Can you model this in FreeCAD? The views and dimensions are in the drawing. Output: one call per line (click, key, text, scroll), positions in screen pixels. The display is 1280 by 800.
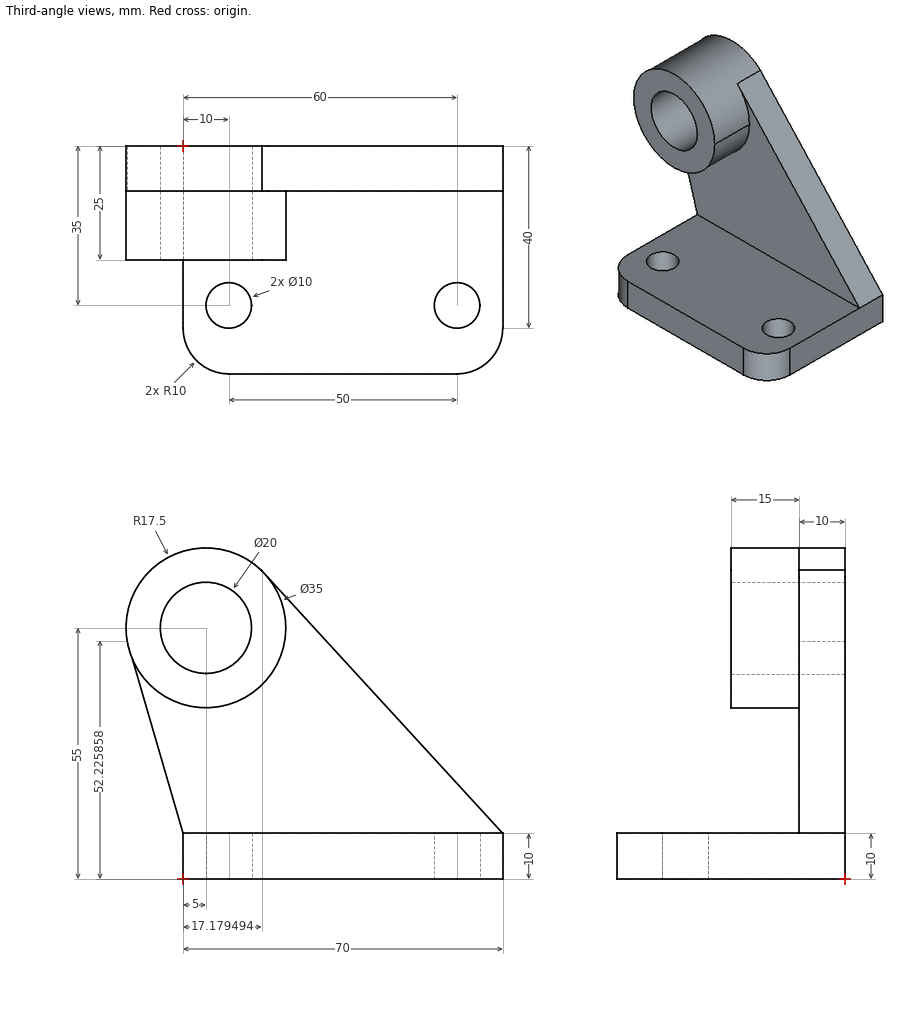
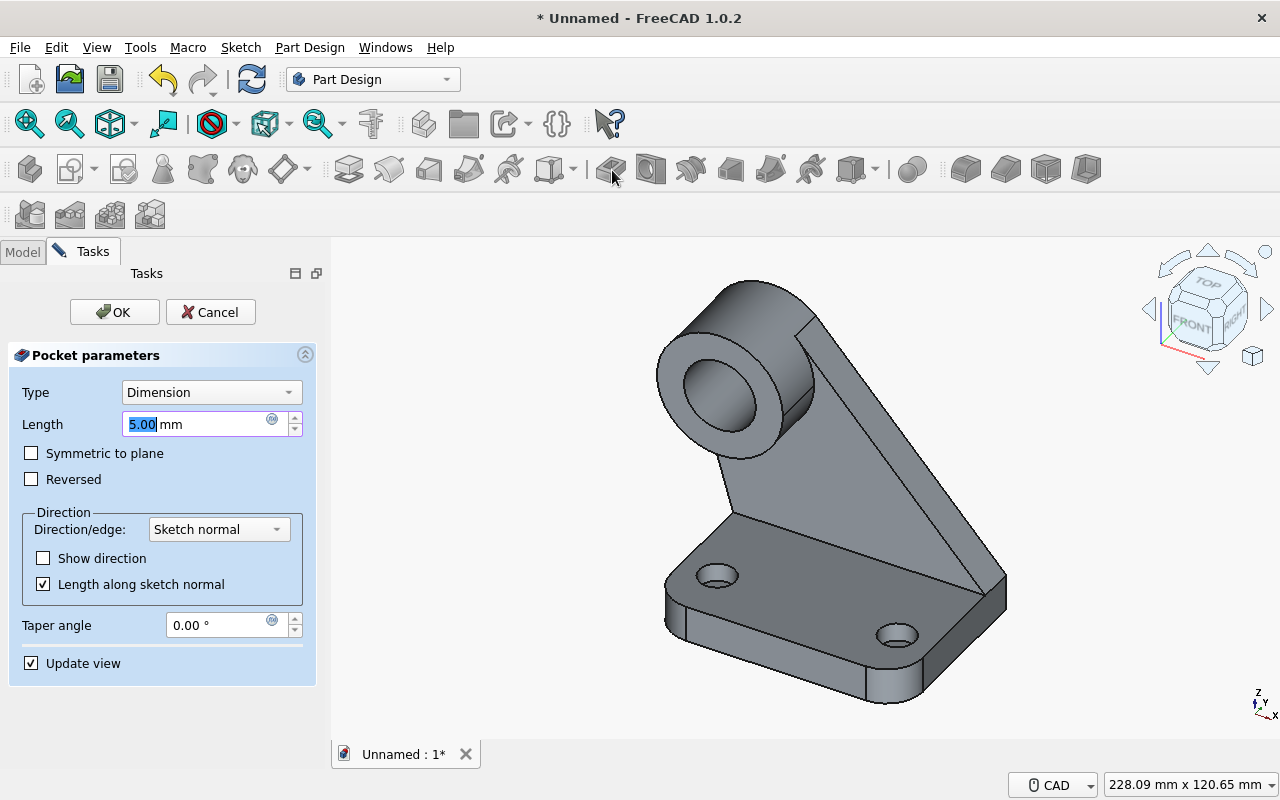
text(10)
key(Tab)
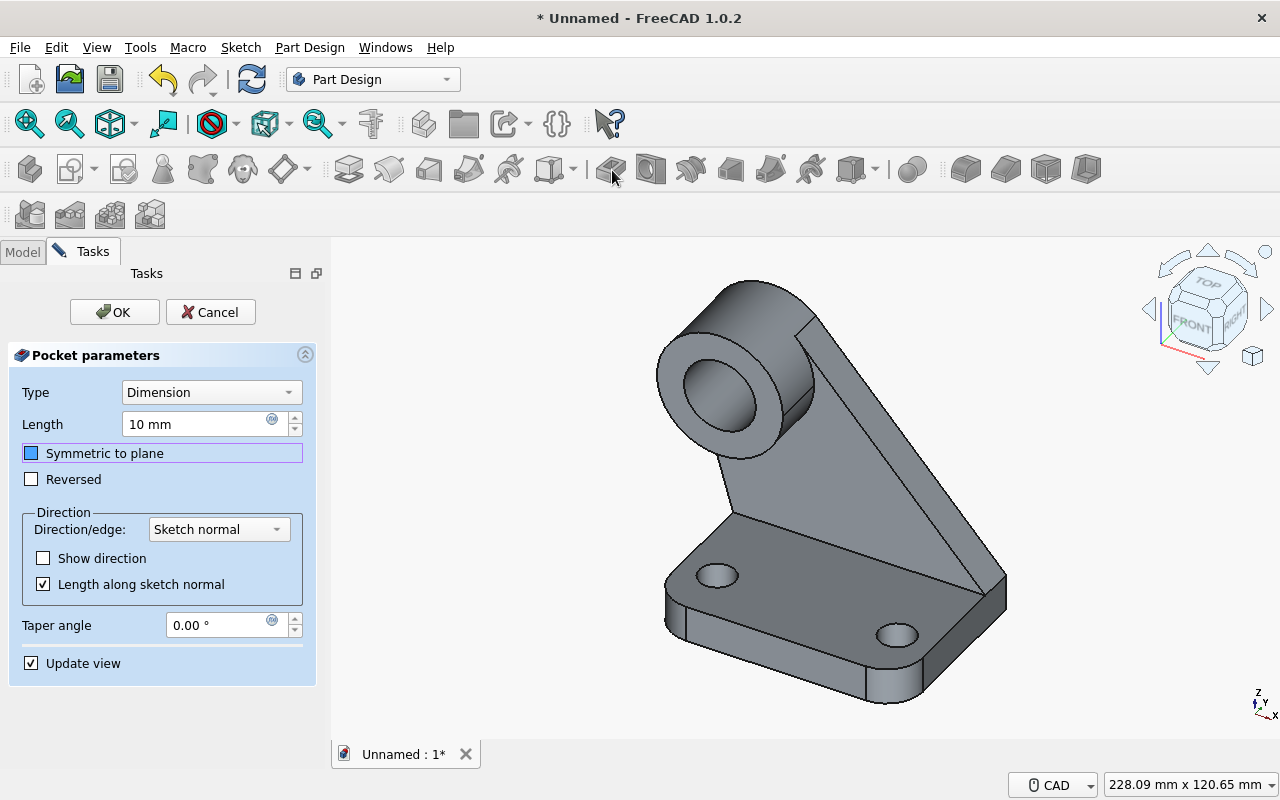
click(115, 312)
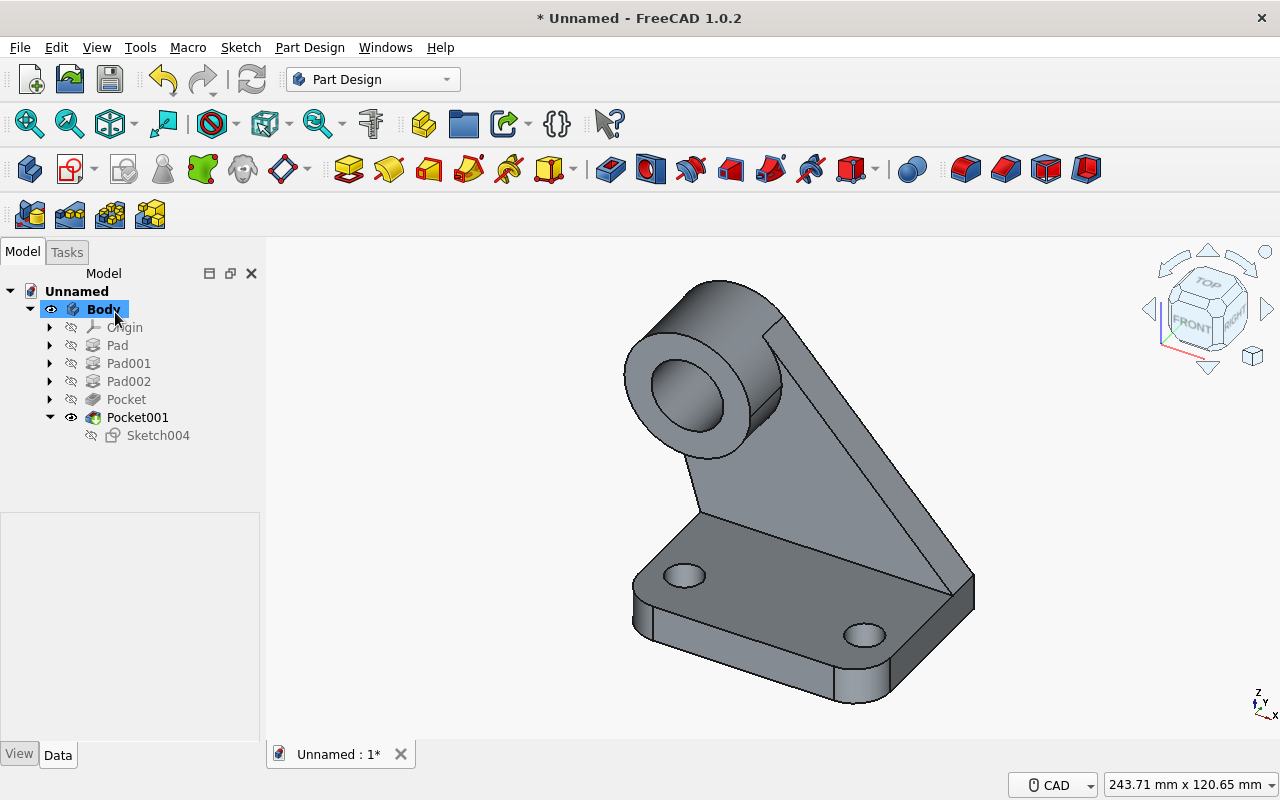
key(0)